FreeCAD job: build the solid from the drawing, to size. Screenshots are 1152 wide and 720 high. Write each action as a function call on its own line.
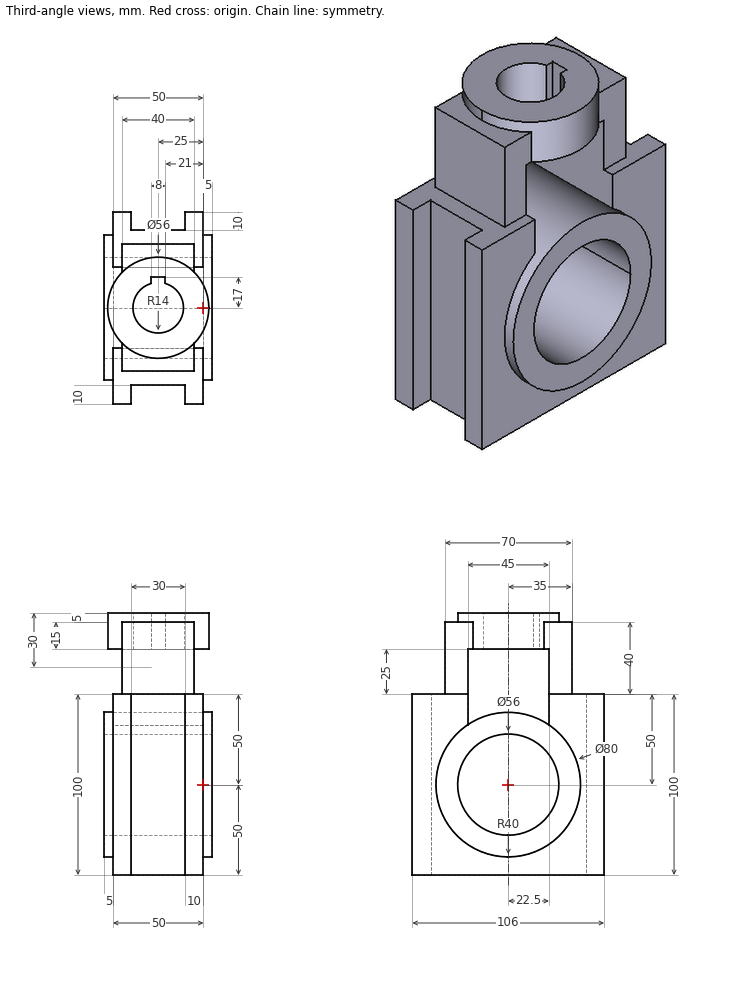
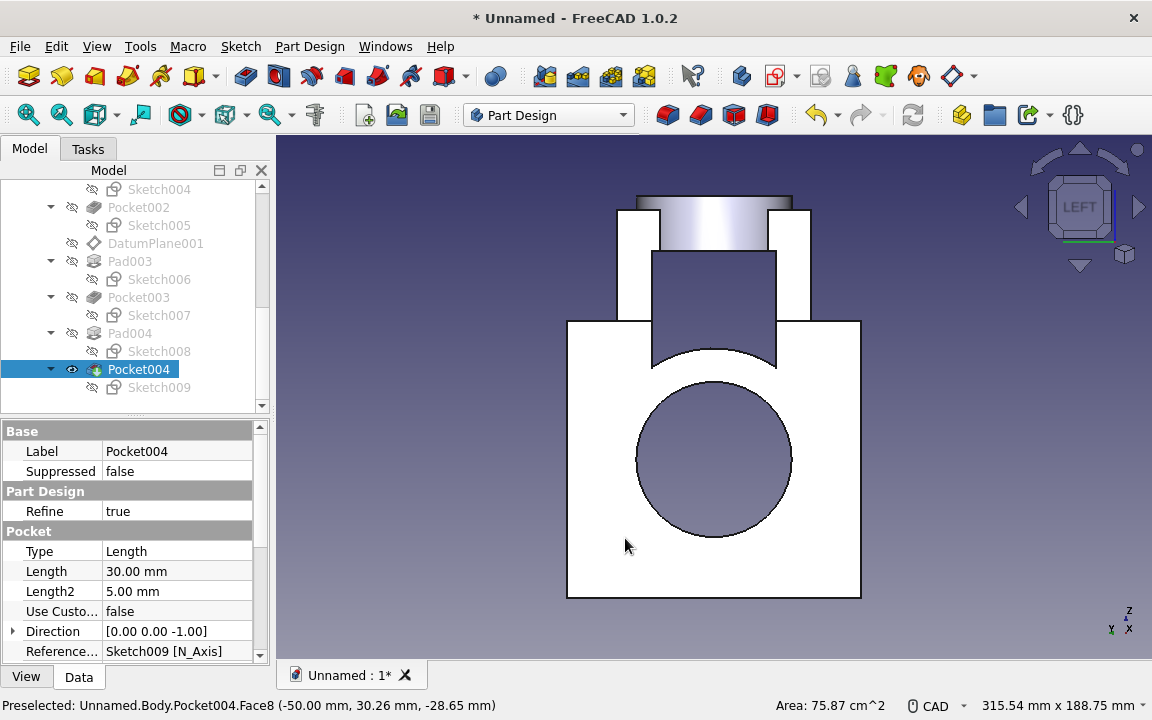
click(774, 76)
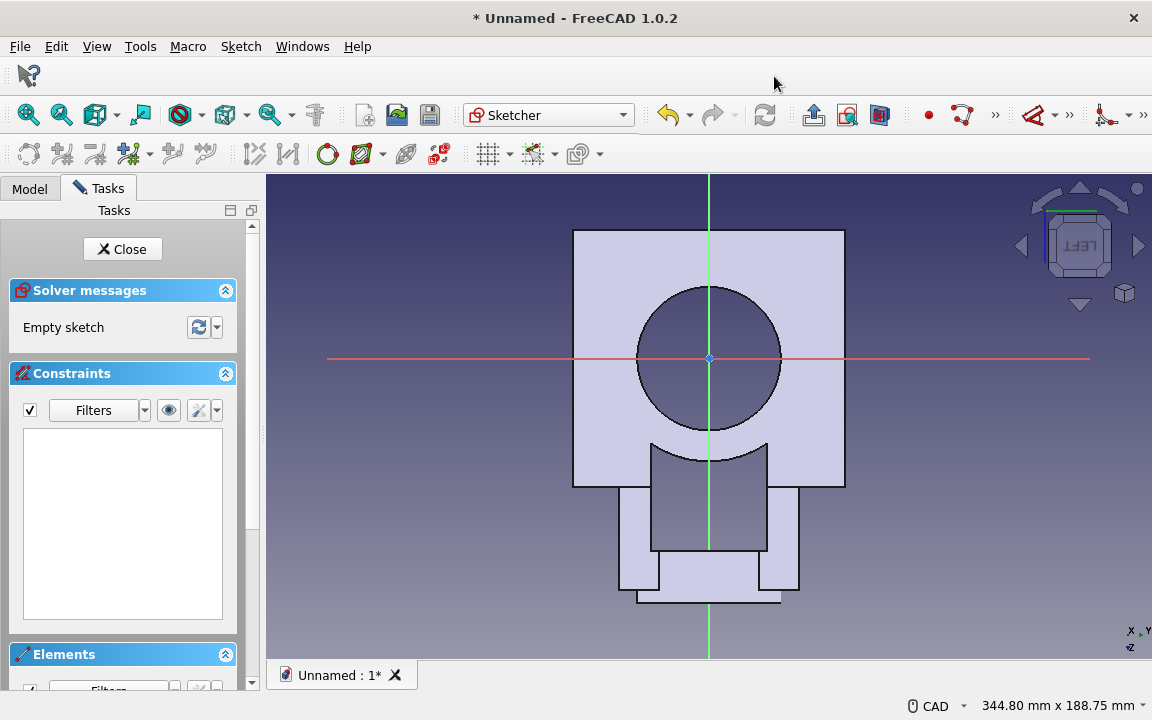
click(880, 116)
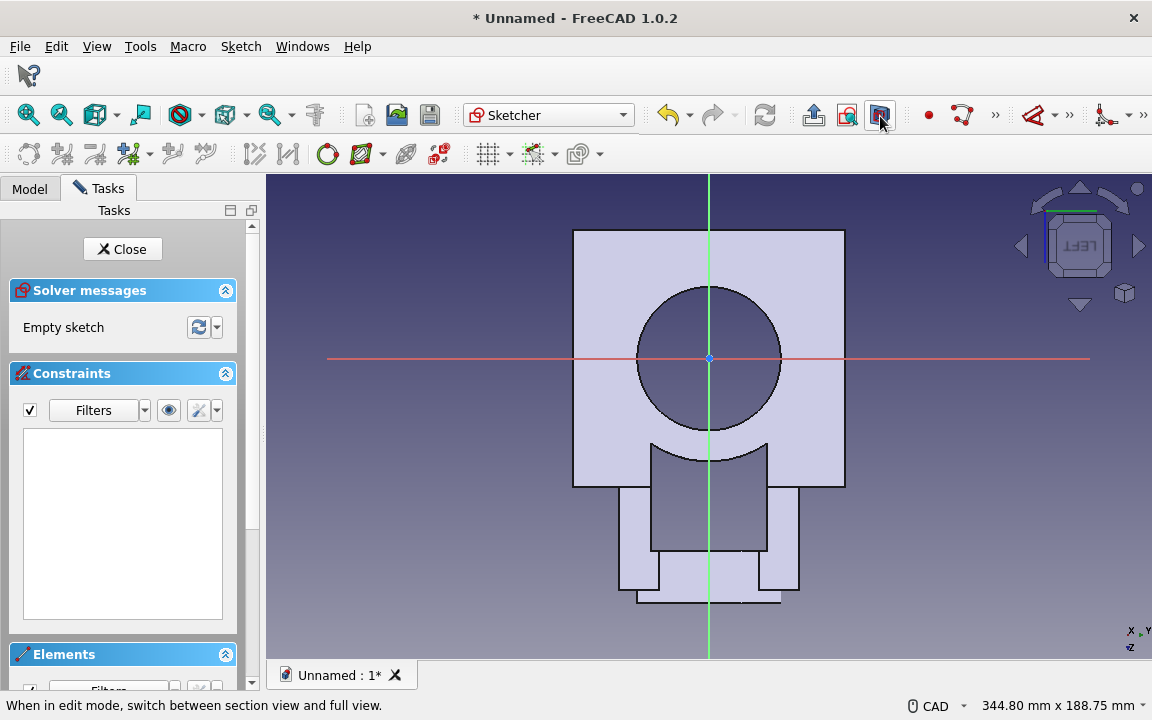
scroll(848, 241, up, 2)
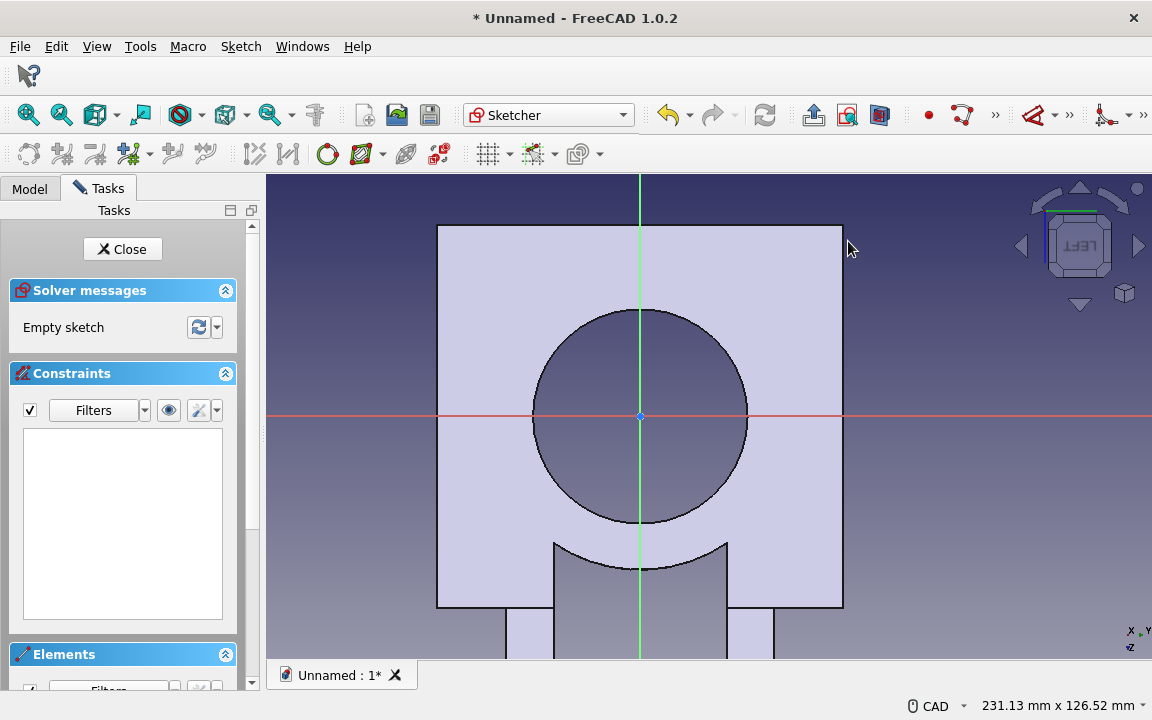
key(g)
key(c)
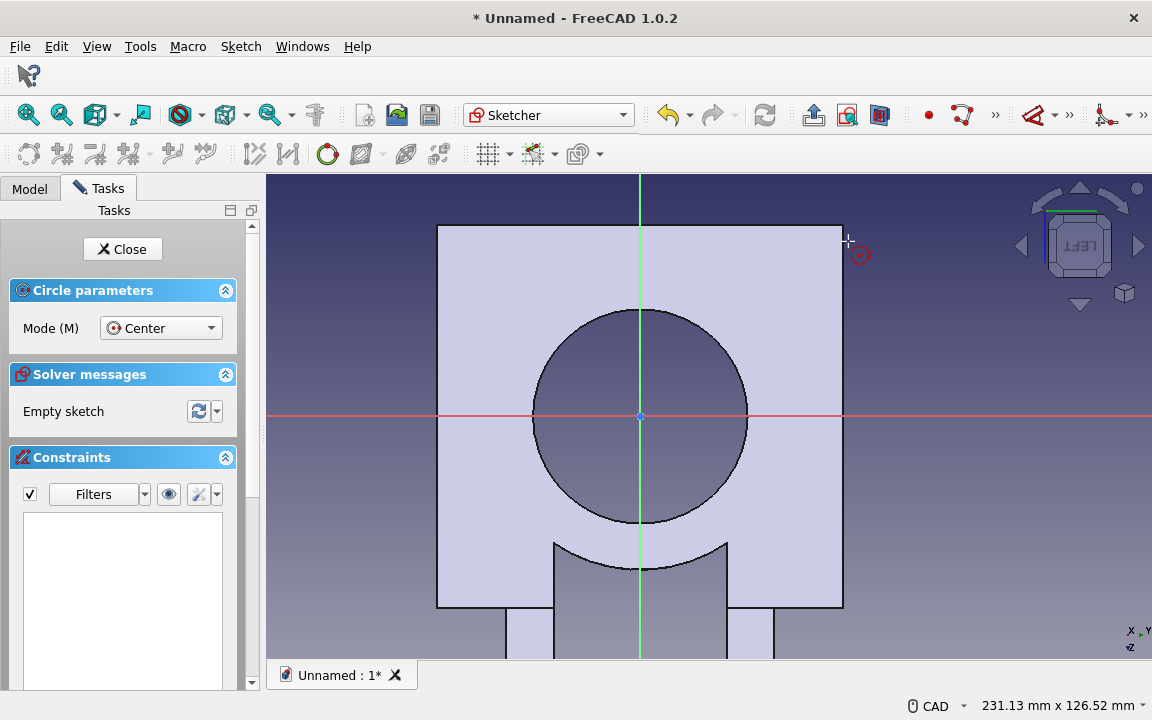
click(640, 416)
move(749, 308)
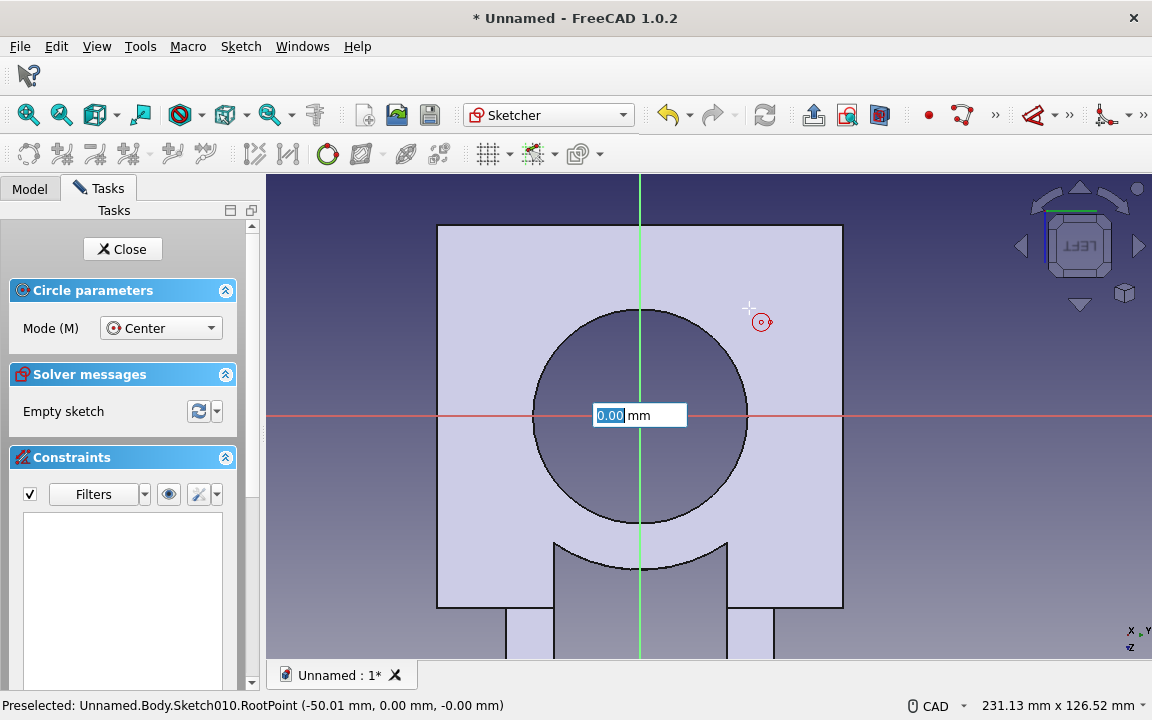
text(80)
key(Return)
key(Escape)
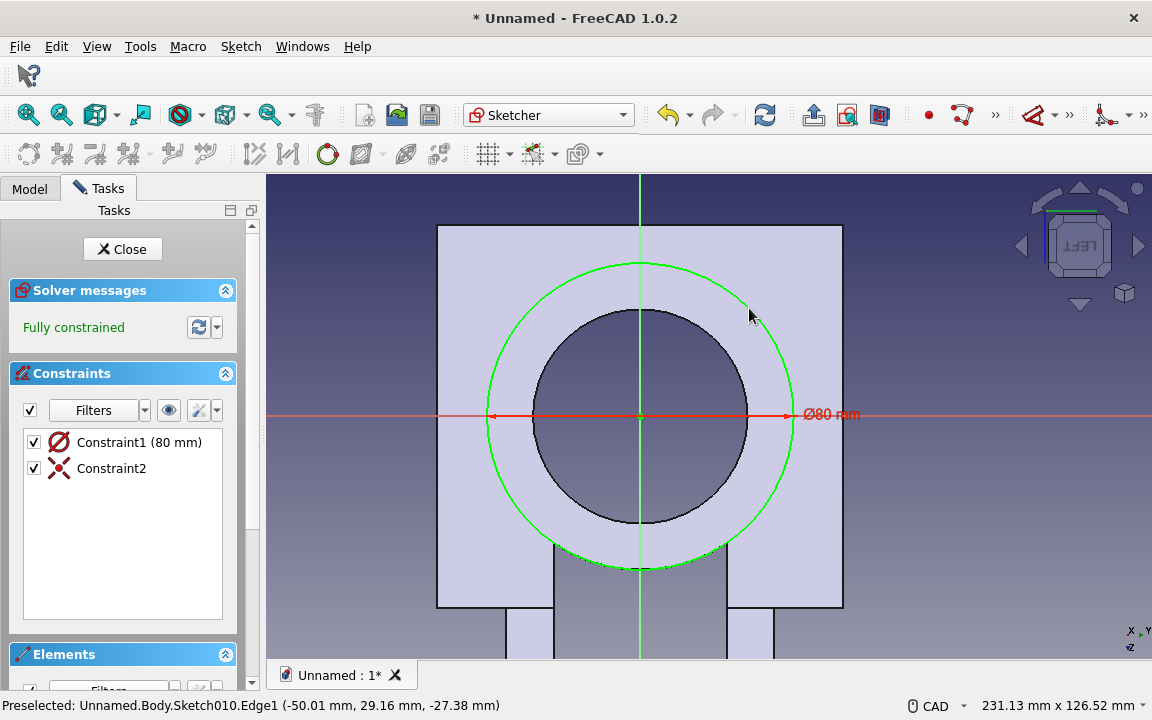
click(123, 249)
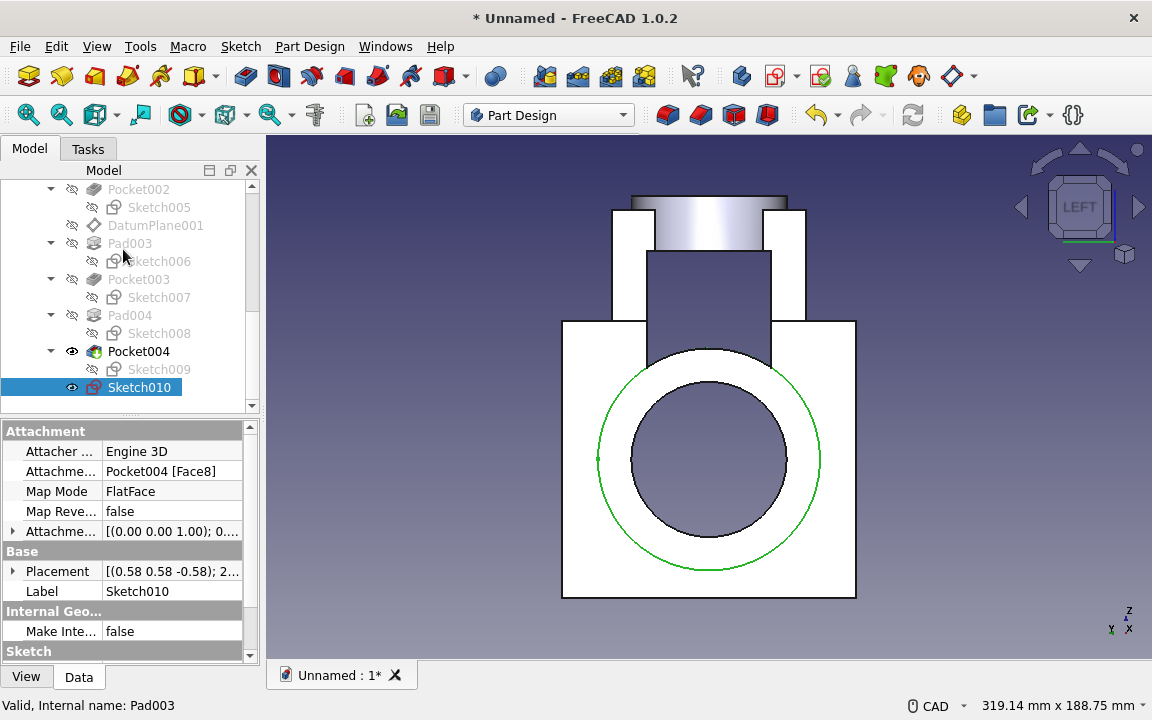
click(29, 76)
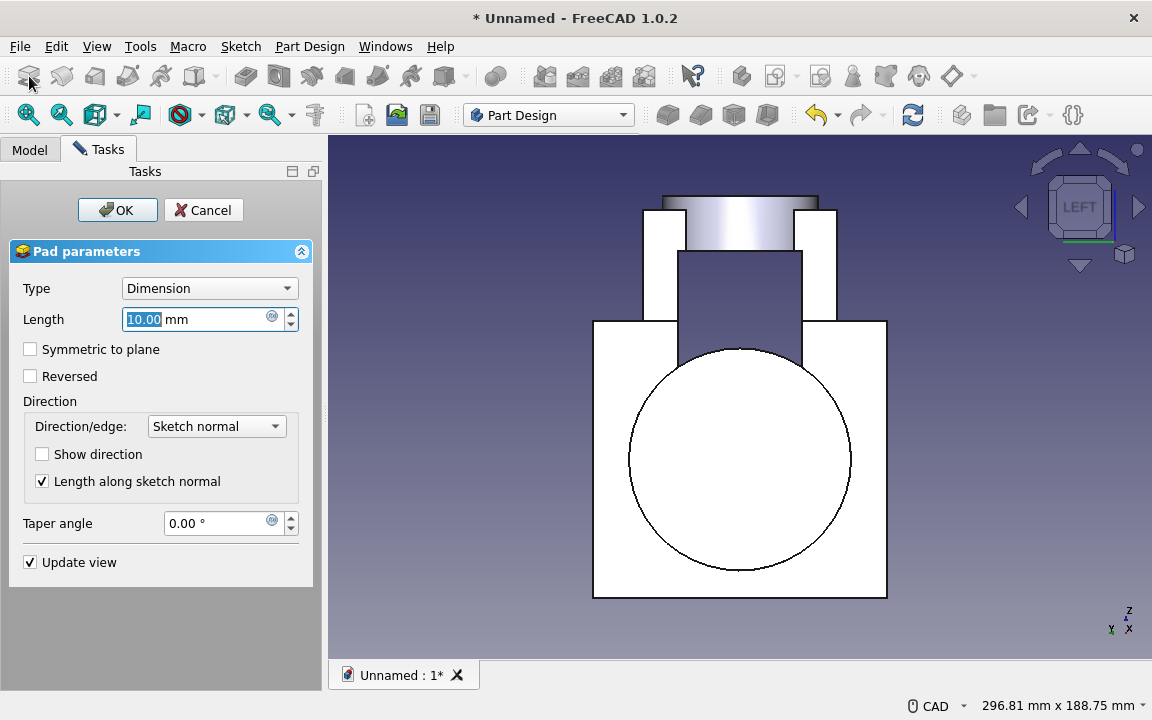
text(5)
key(Tab)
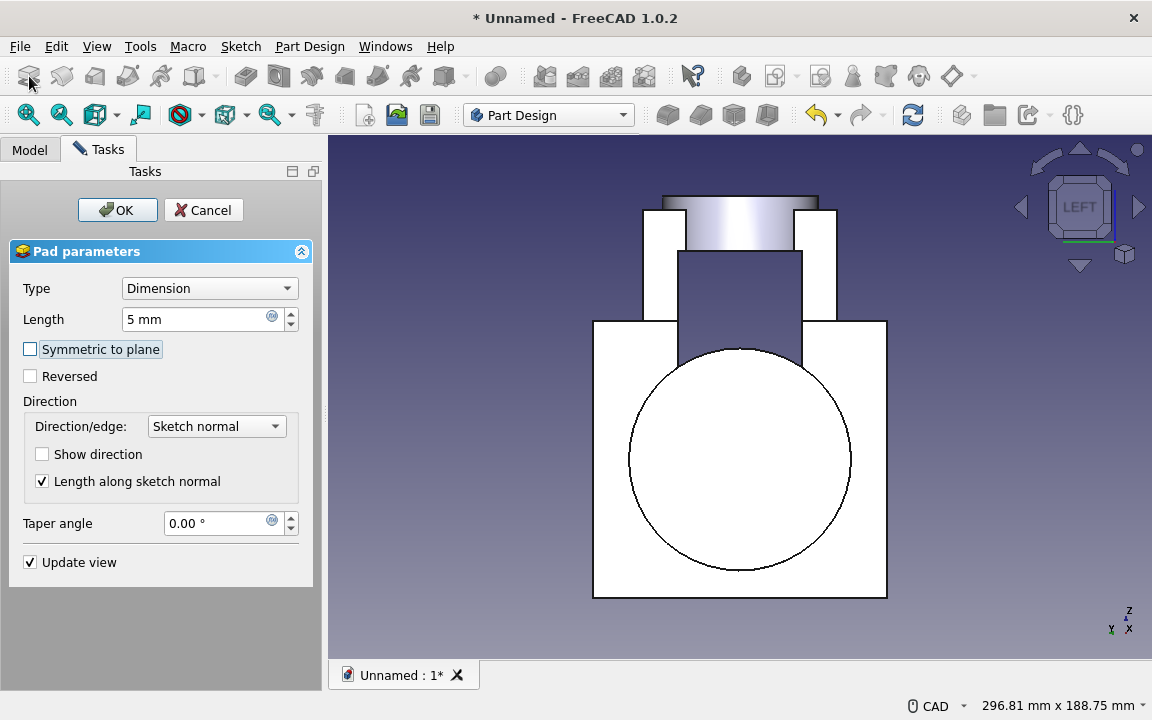
click(118, 210)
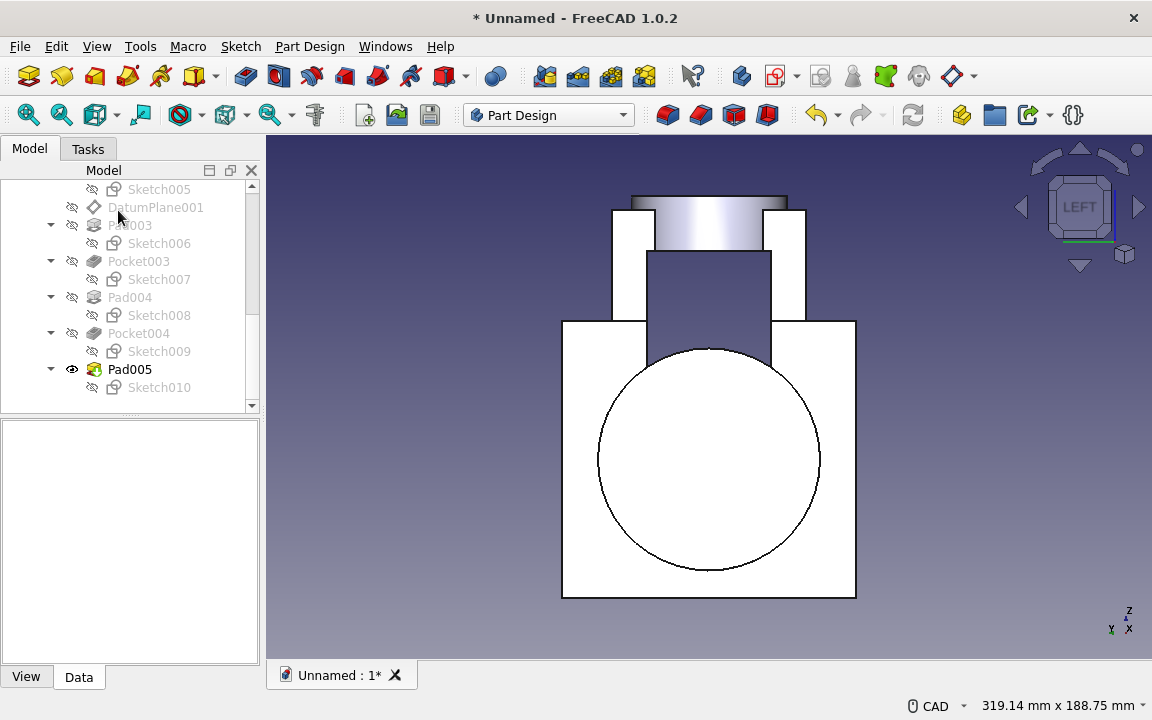
key(0)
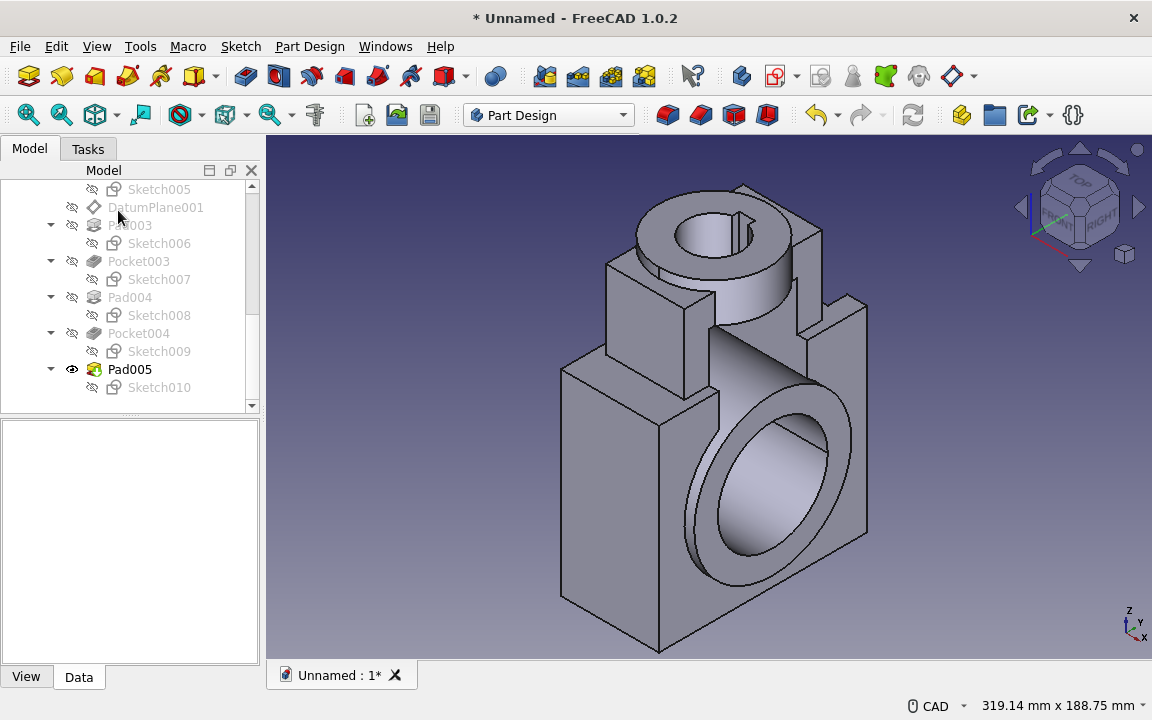
click(840, 445)